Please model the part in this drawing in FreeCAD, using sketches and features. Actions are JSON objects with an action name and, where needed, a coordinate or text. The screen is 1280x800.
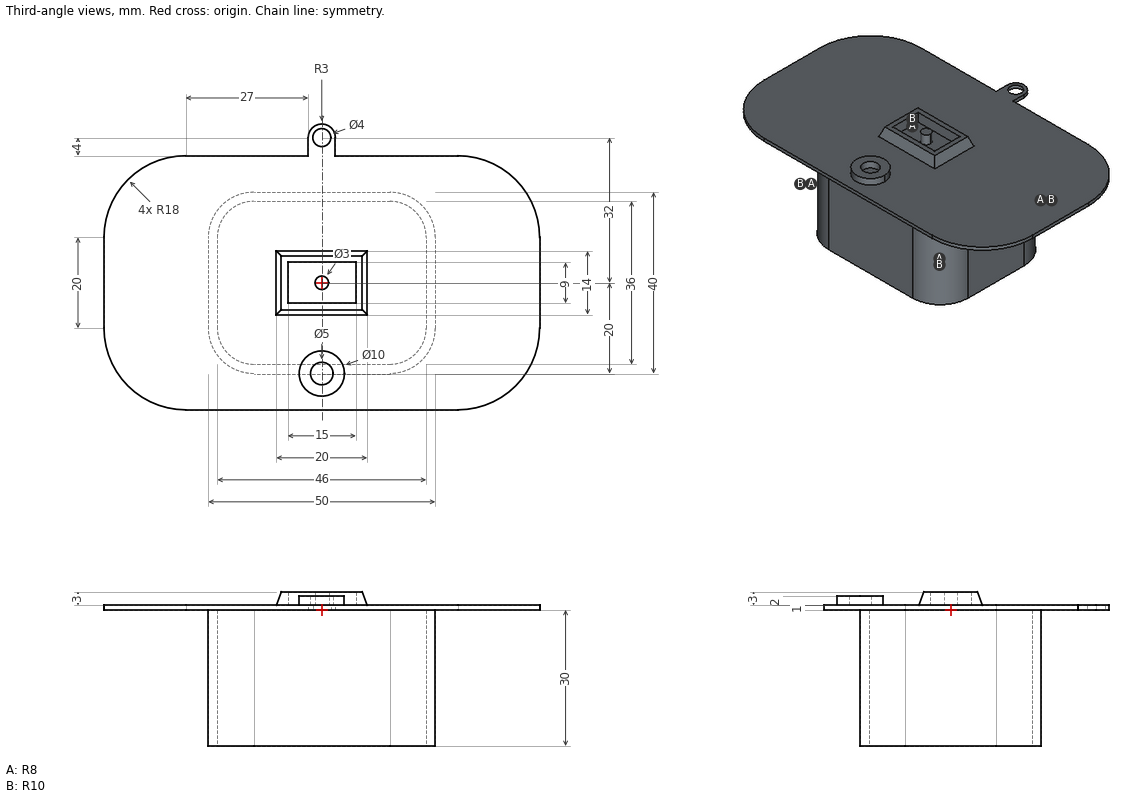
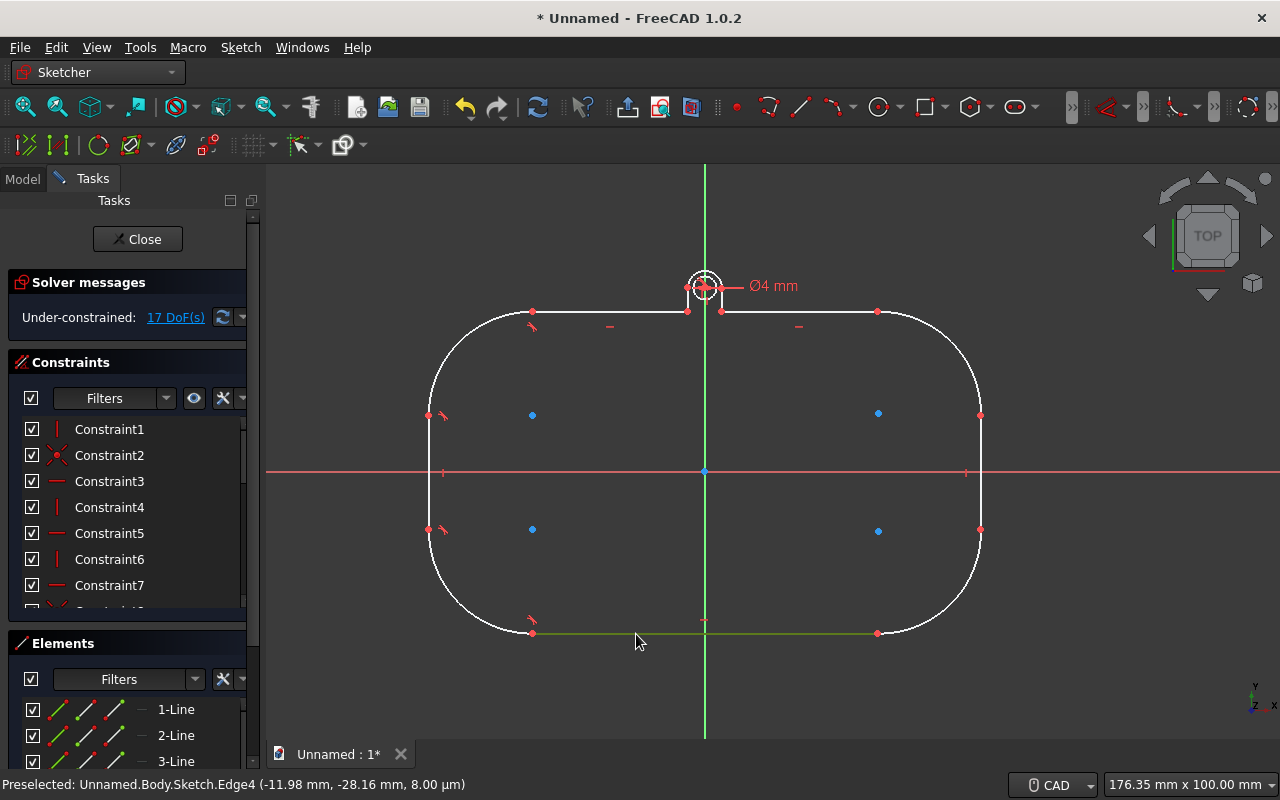
{"action": "left_click", "coordinate": [925, 623]}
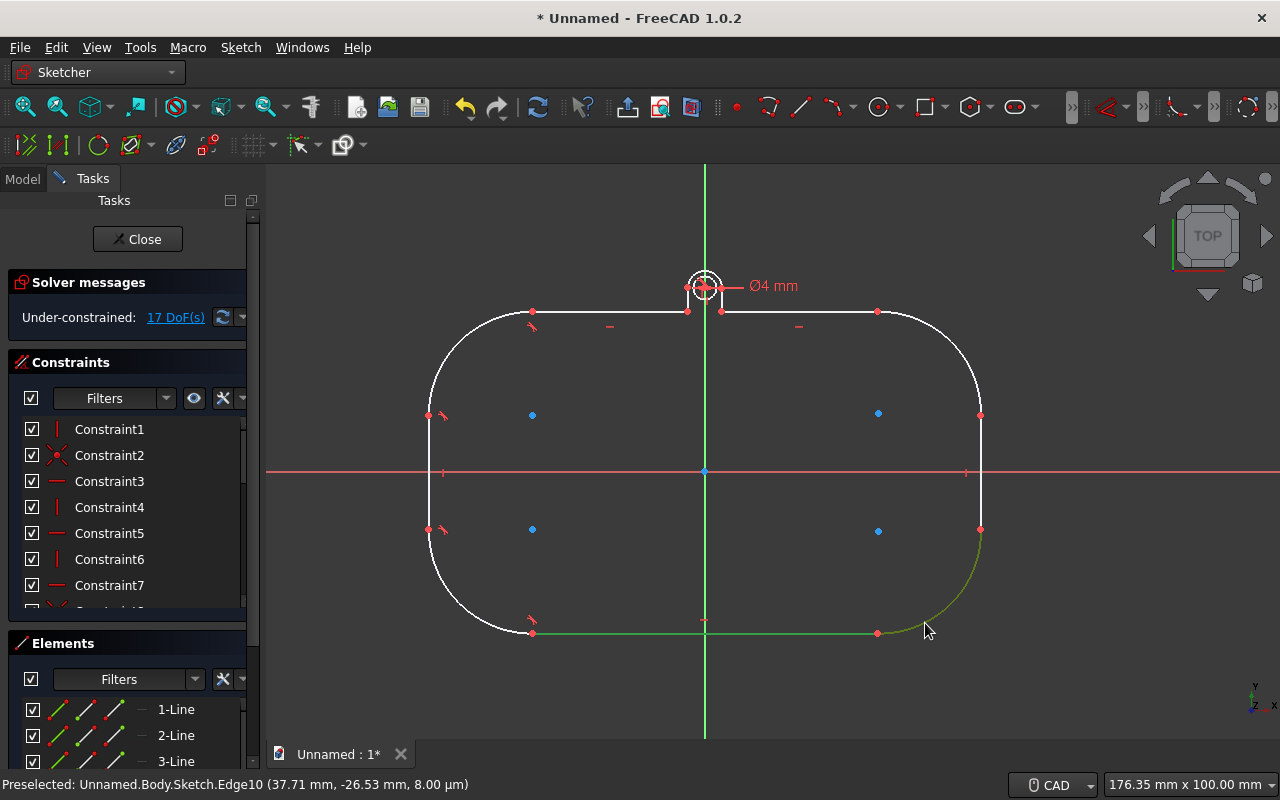
{"action": "key", "text": "t"}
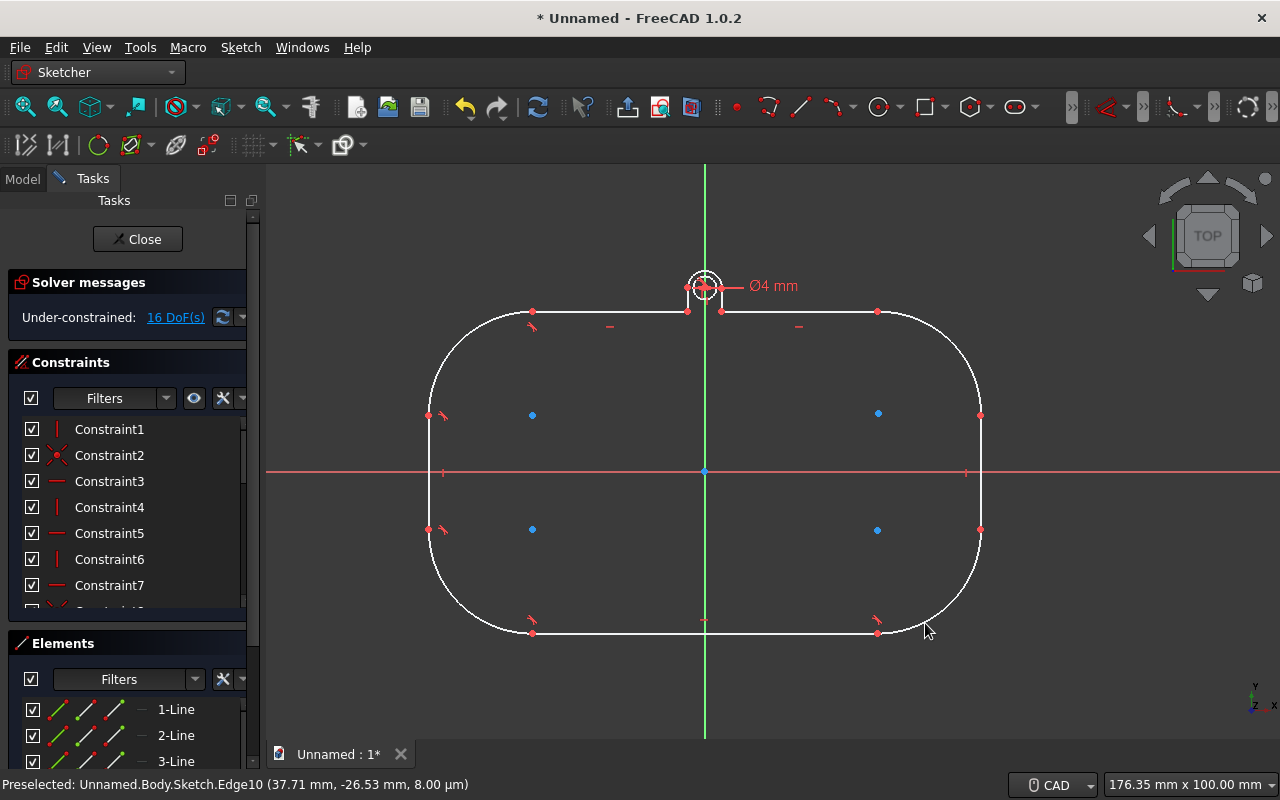
{"action": "left_click", "coordinate": [981, 496]}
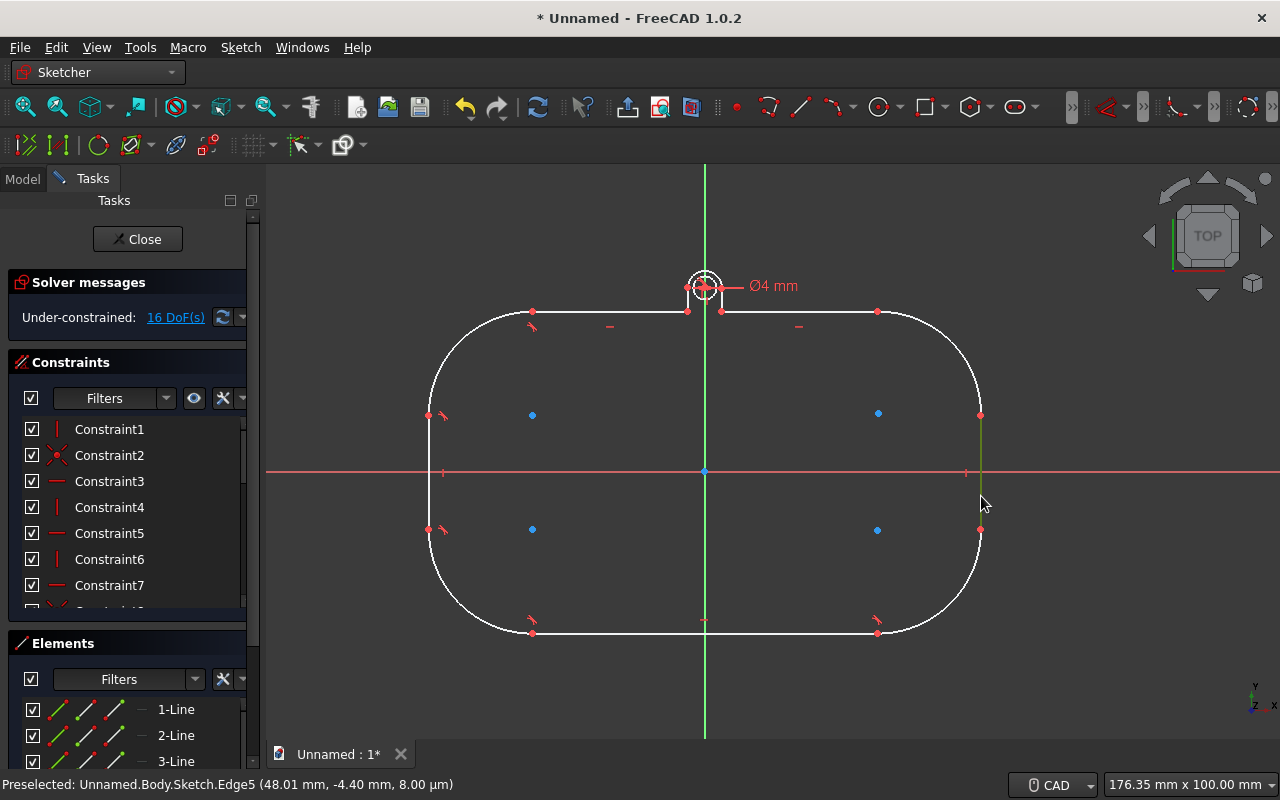
{"action": "left_click", "coordinate": [924, 622]}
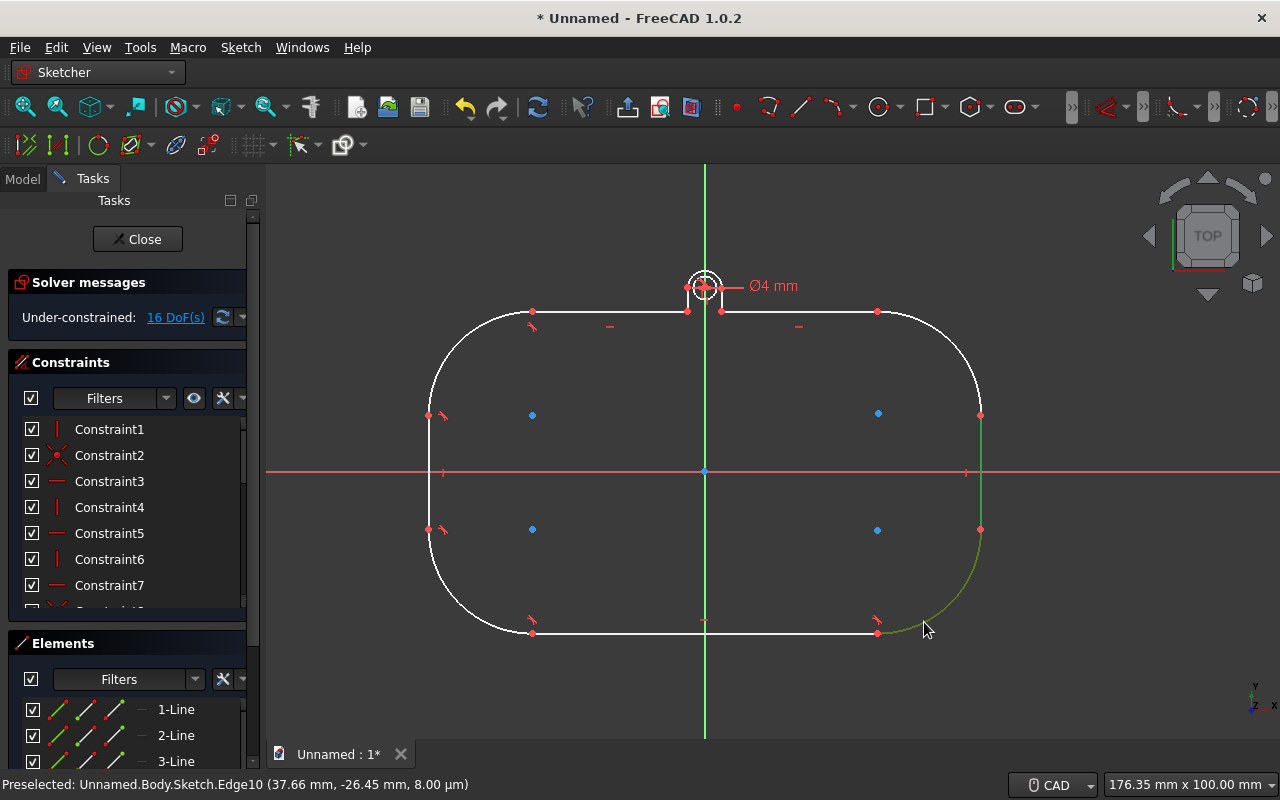
{"action": "key", "text": "t"}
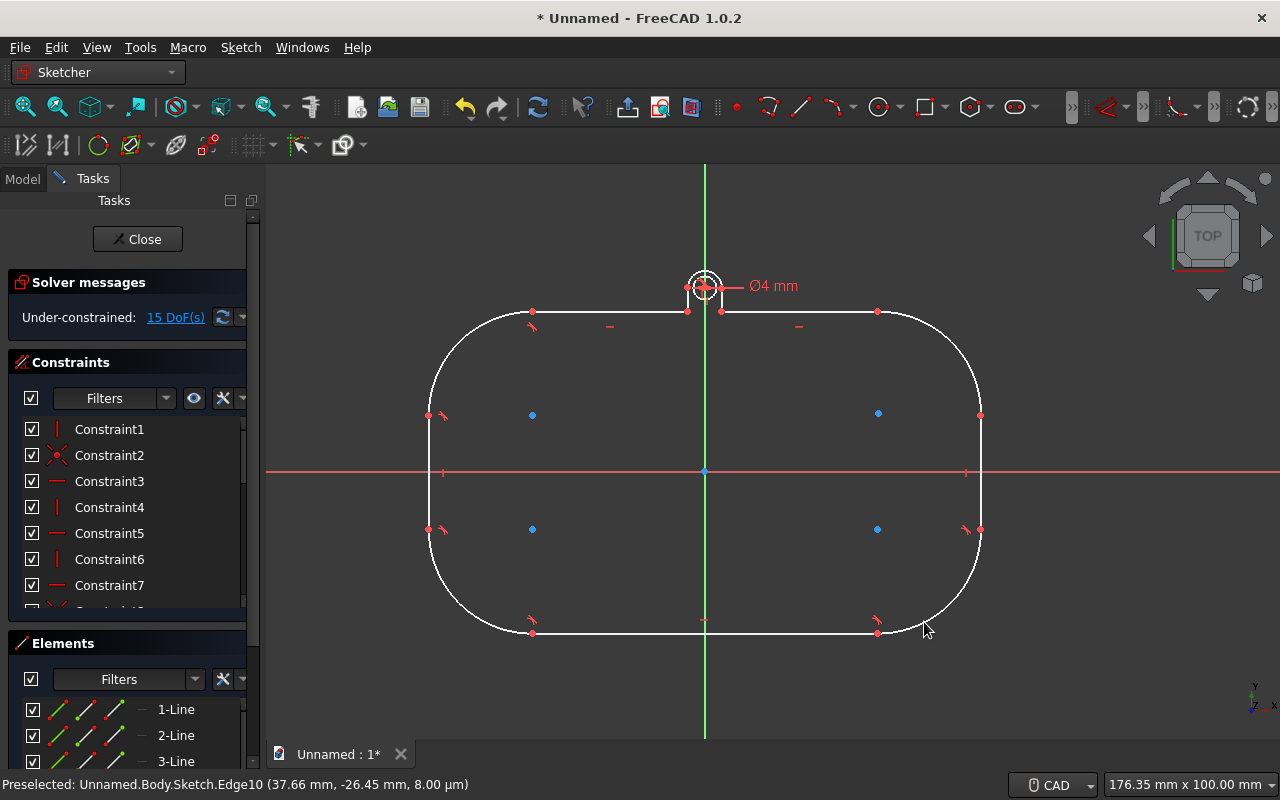
{"action": "left_click", "coordinate": [981, 496]}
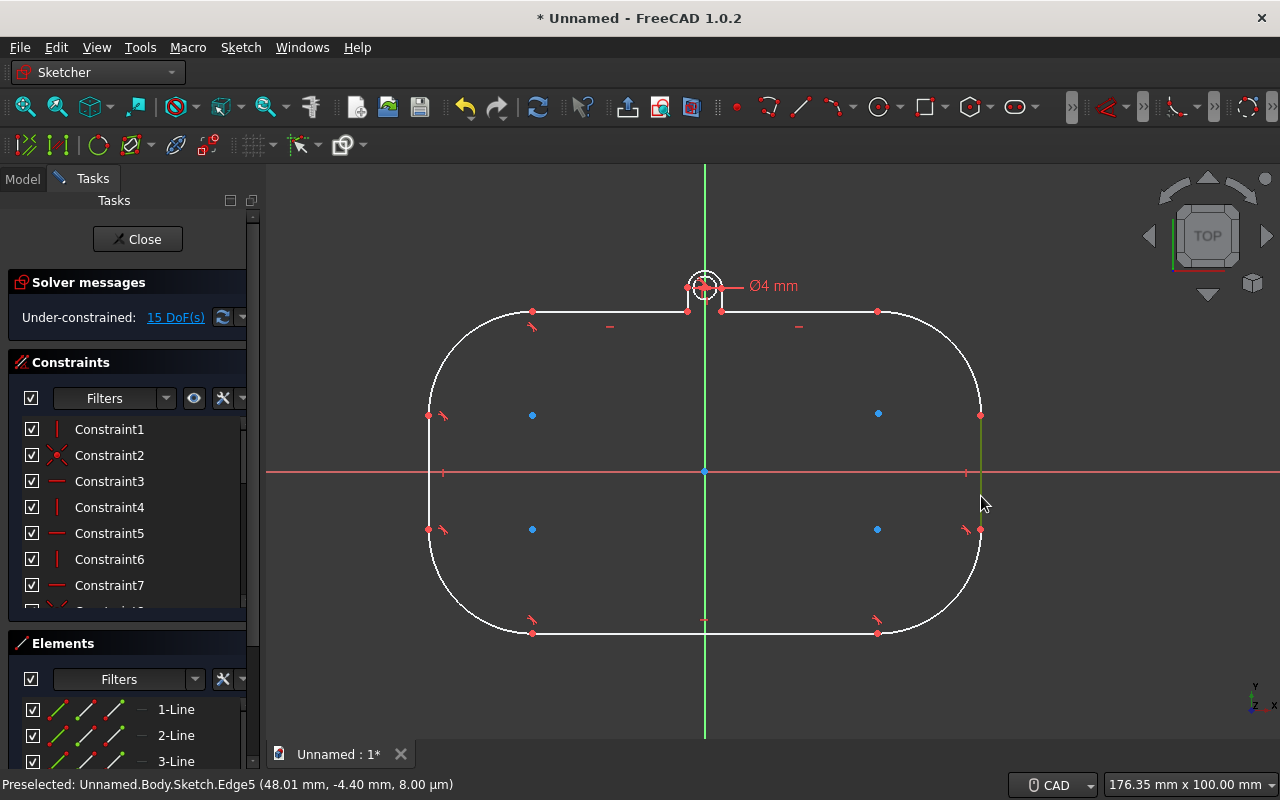
{"action": "left_click", "coordinate": [970, 368]}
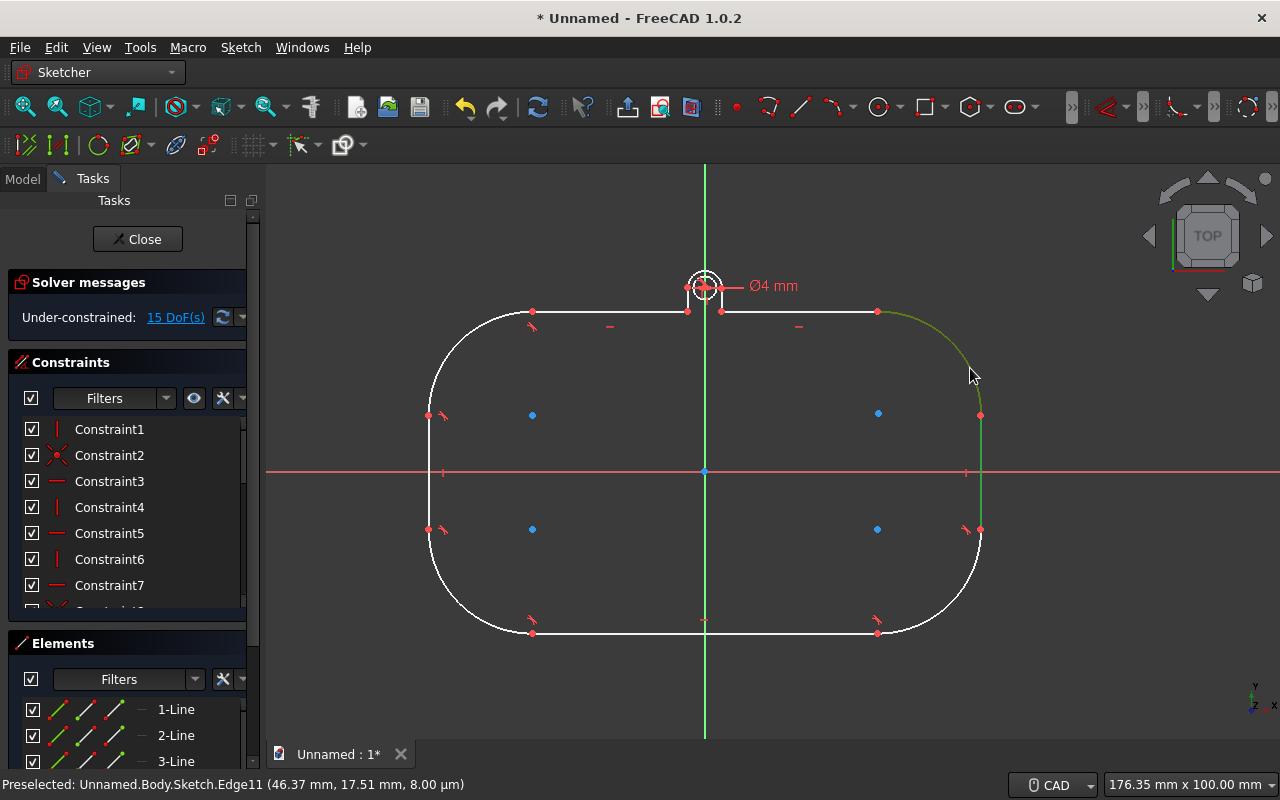
{"action": "key", "text": "t"}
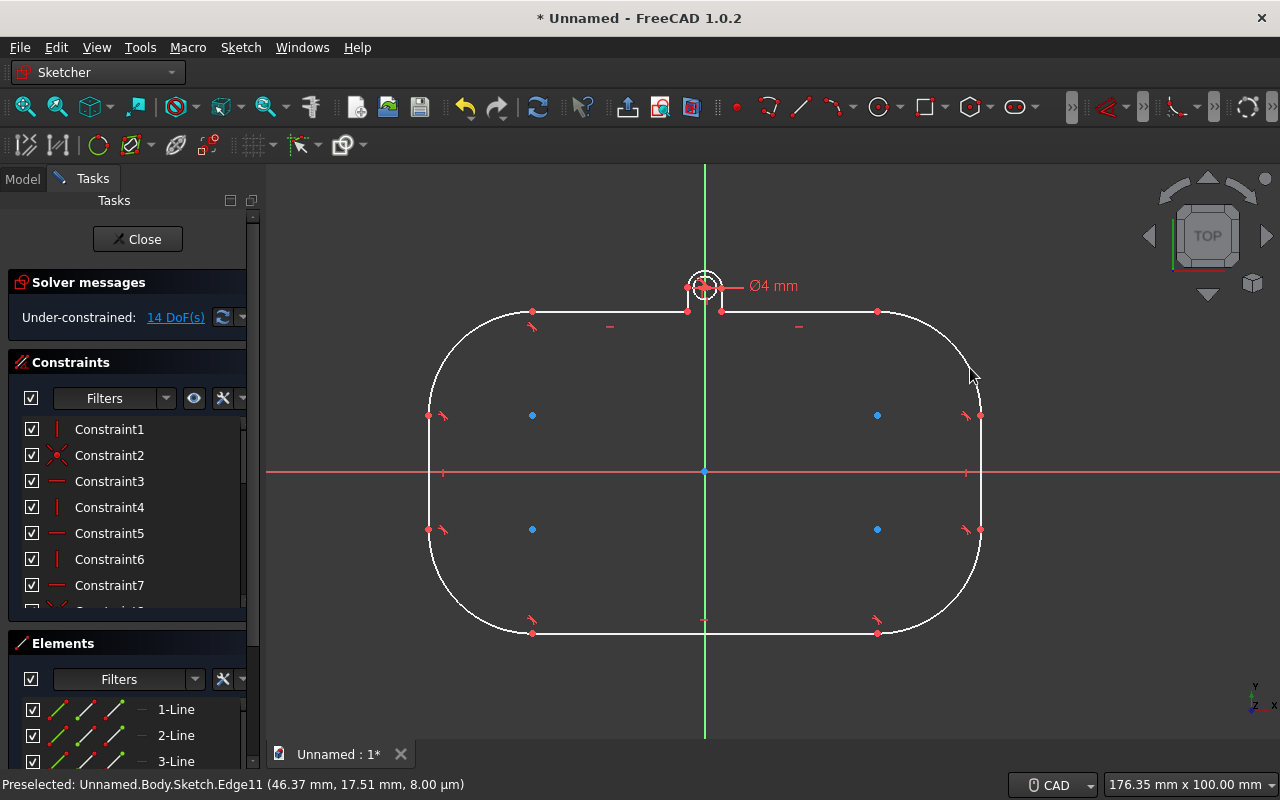
{"action": "left_click", "coordinate": [831, 312]}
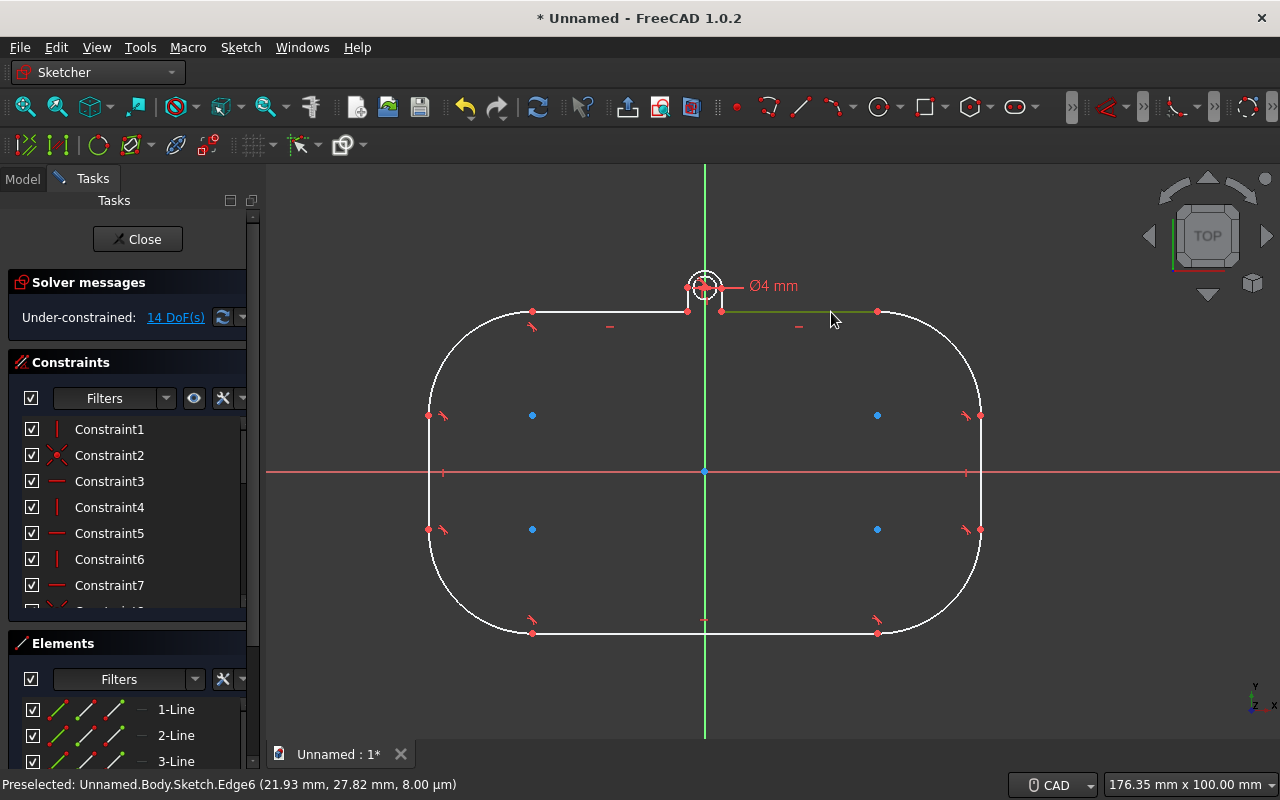
{"action": "left_click", "coordinate": [970, 368]}